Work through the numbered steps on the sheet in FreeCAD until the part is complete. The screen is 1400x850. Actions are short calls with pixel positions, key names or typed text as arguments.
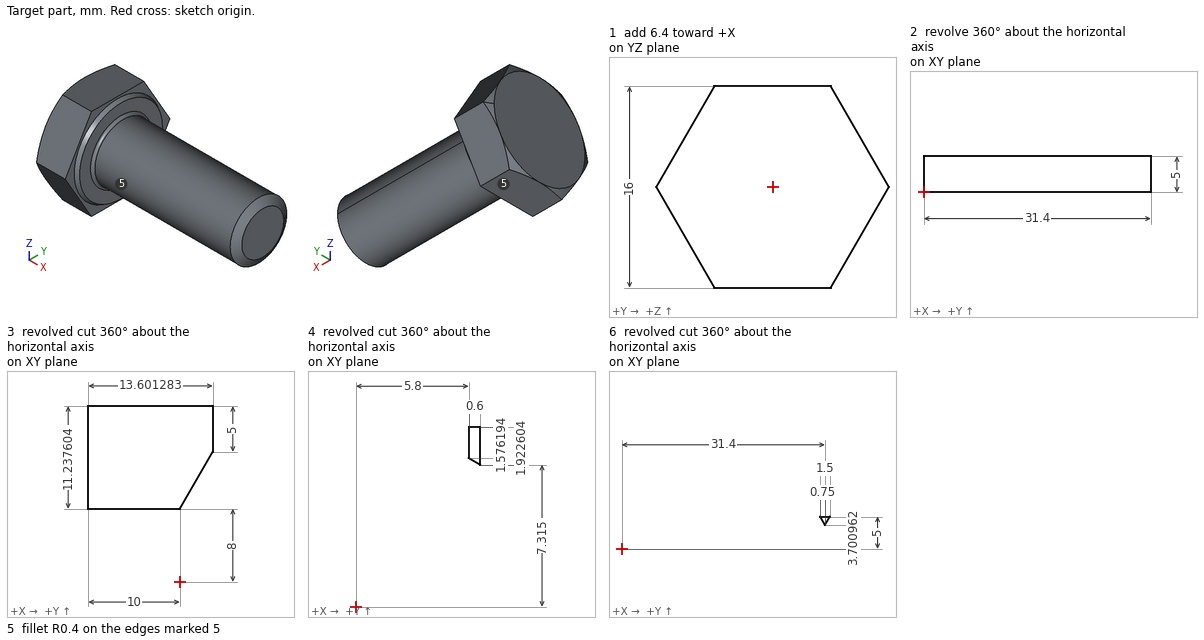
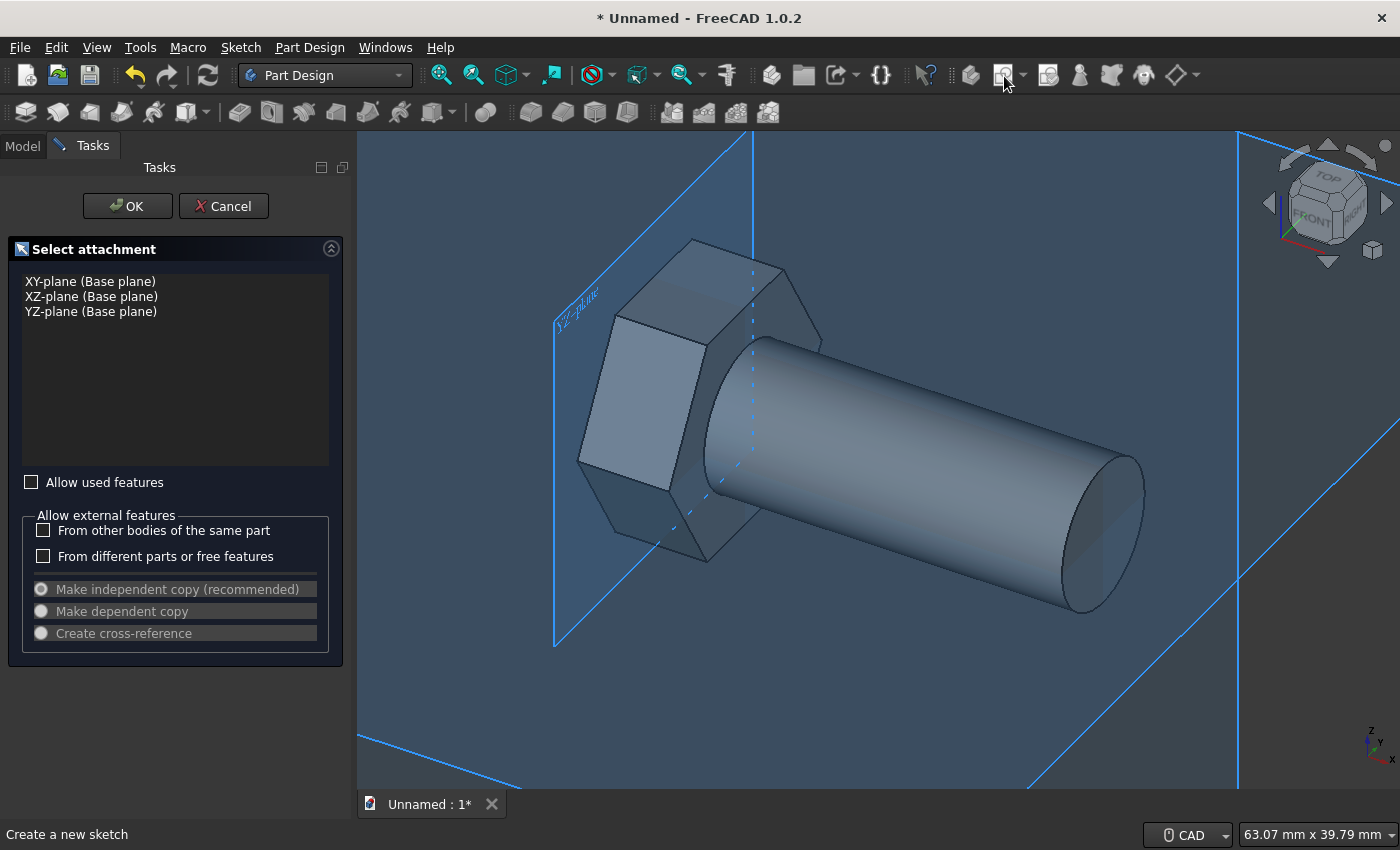
click(82, 282)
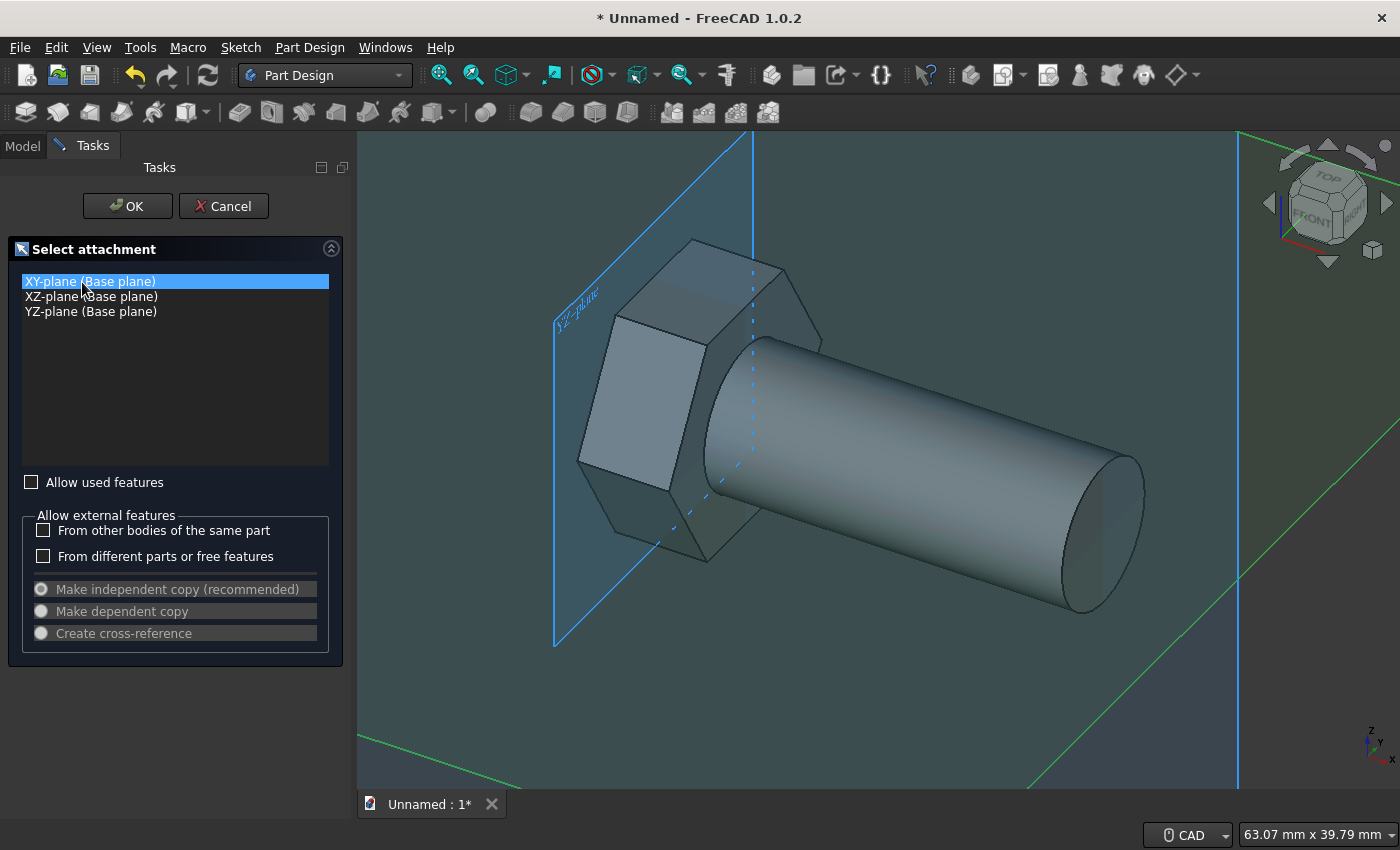
click(128, 206)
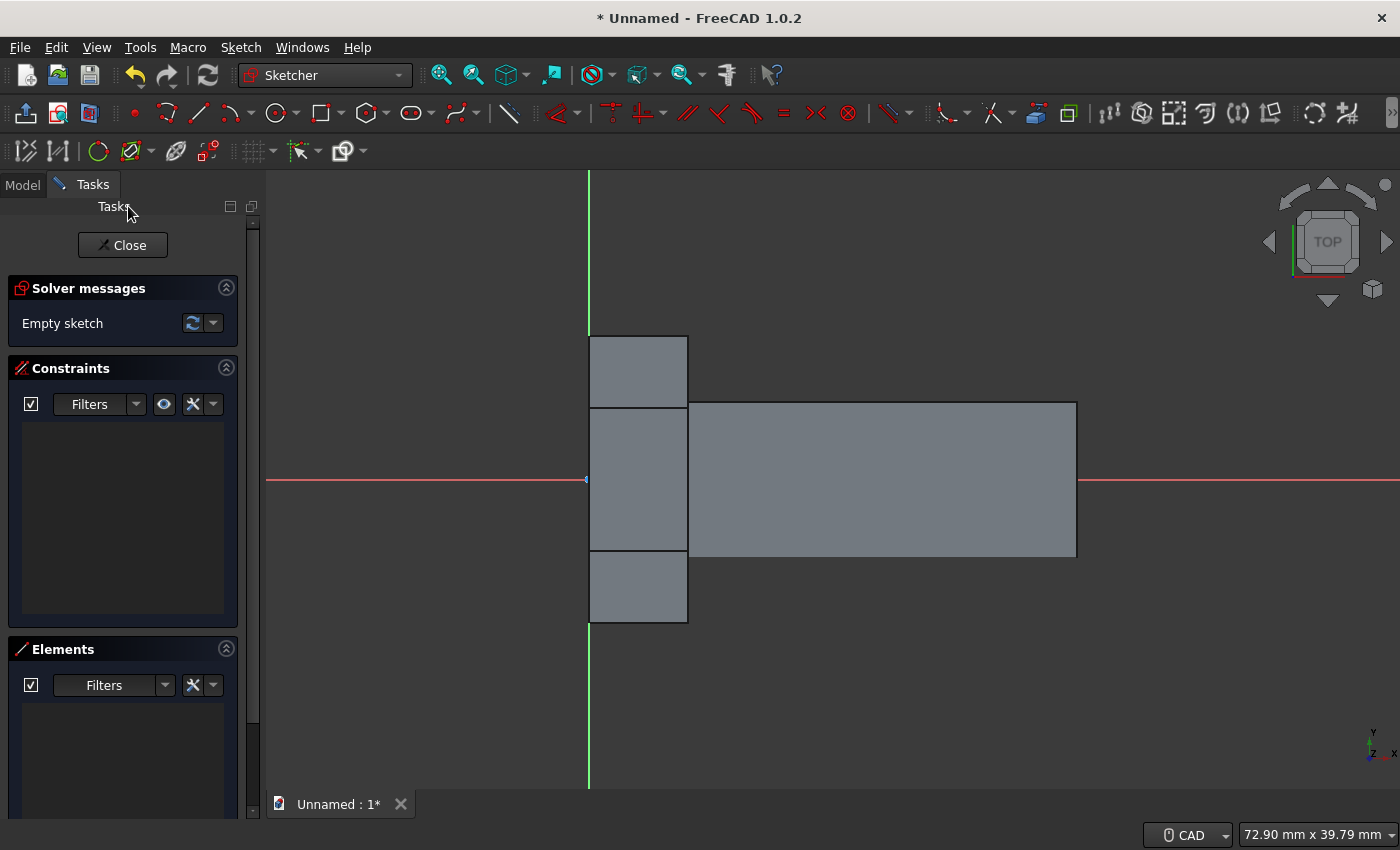
key(q)
key(s)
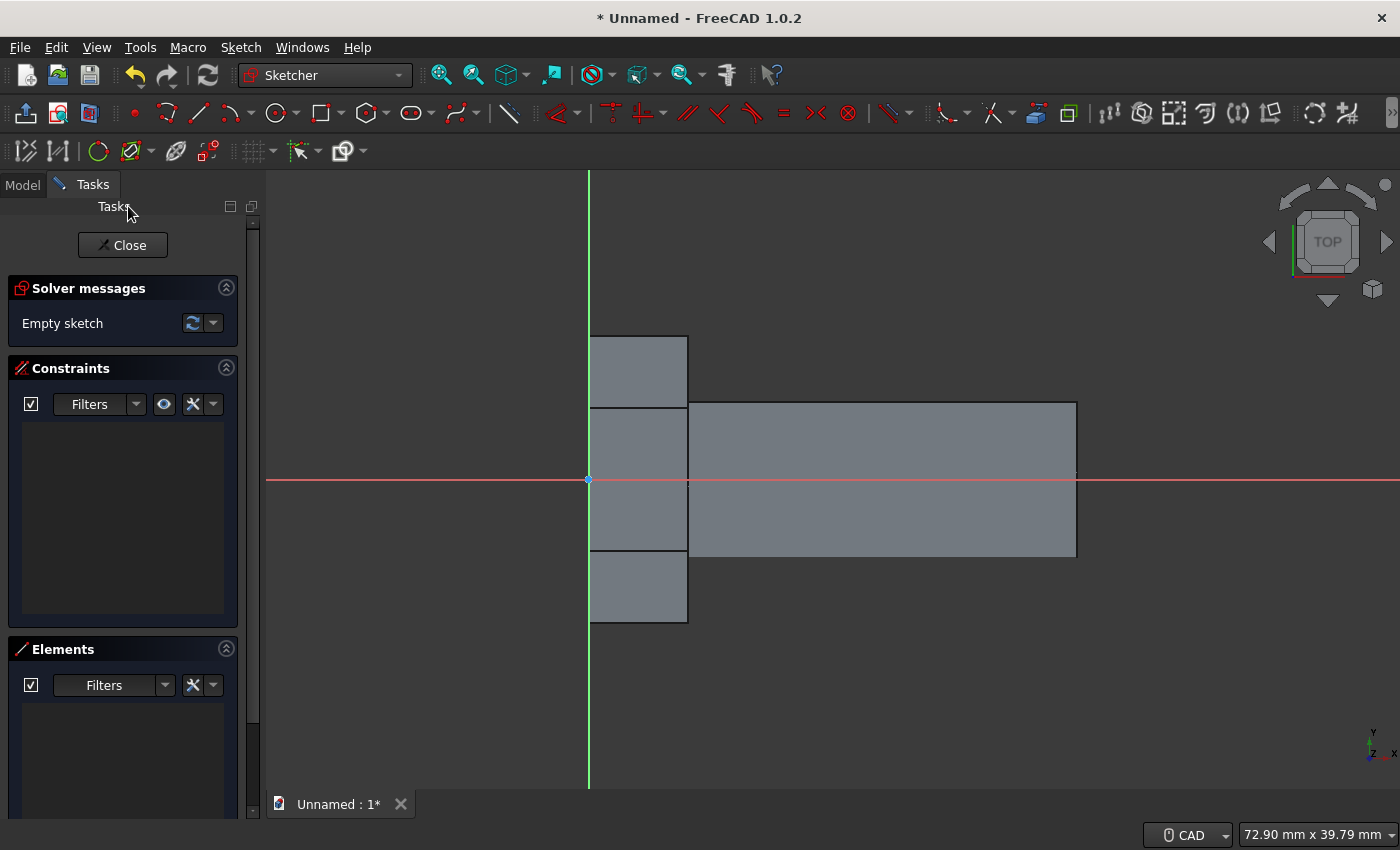
scroll(1235, 761, down, 1)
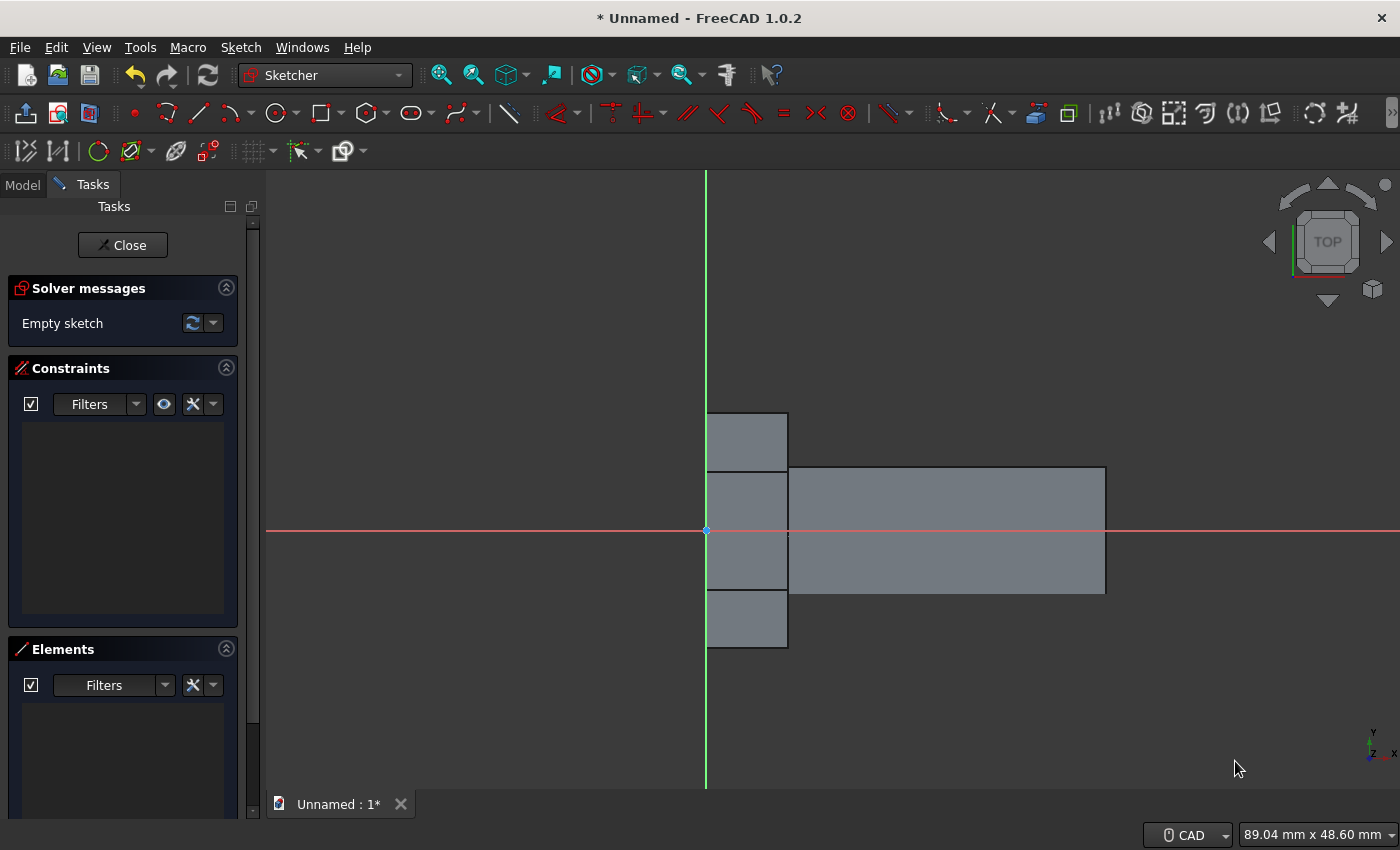
scroll(464, 263, up, 2)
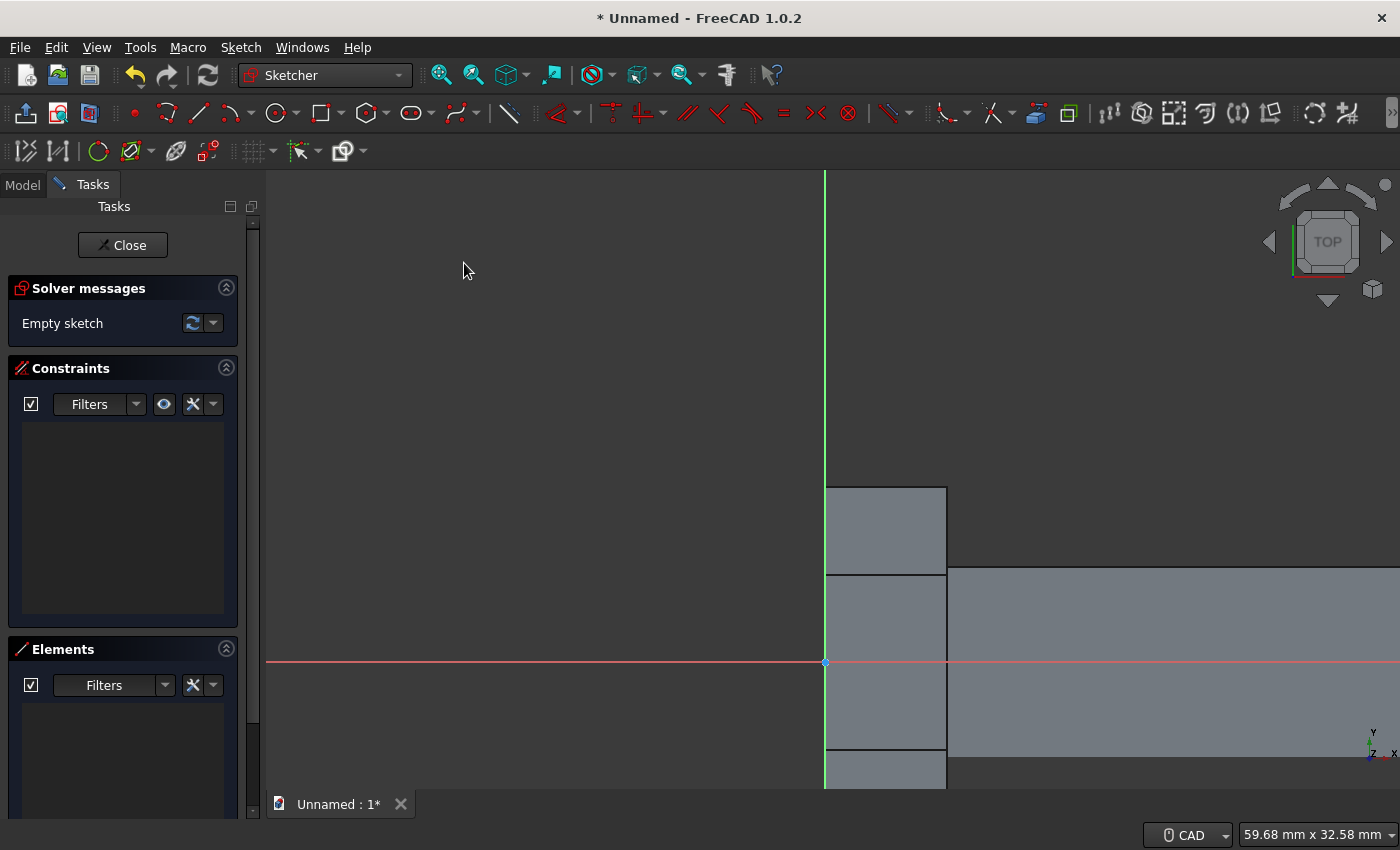
click(168, 114)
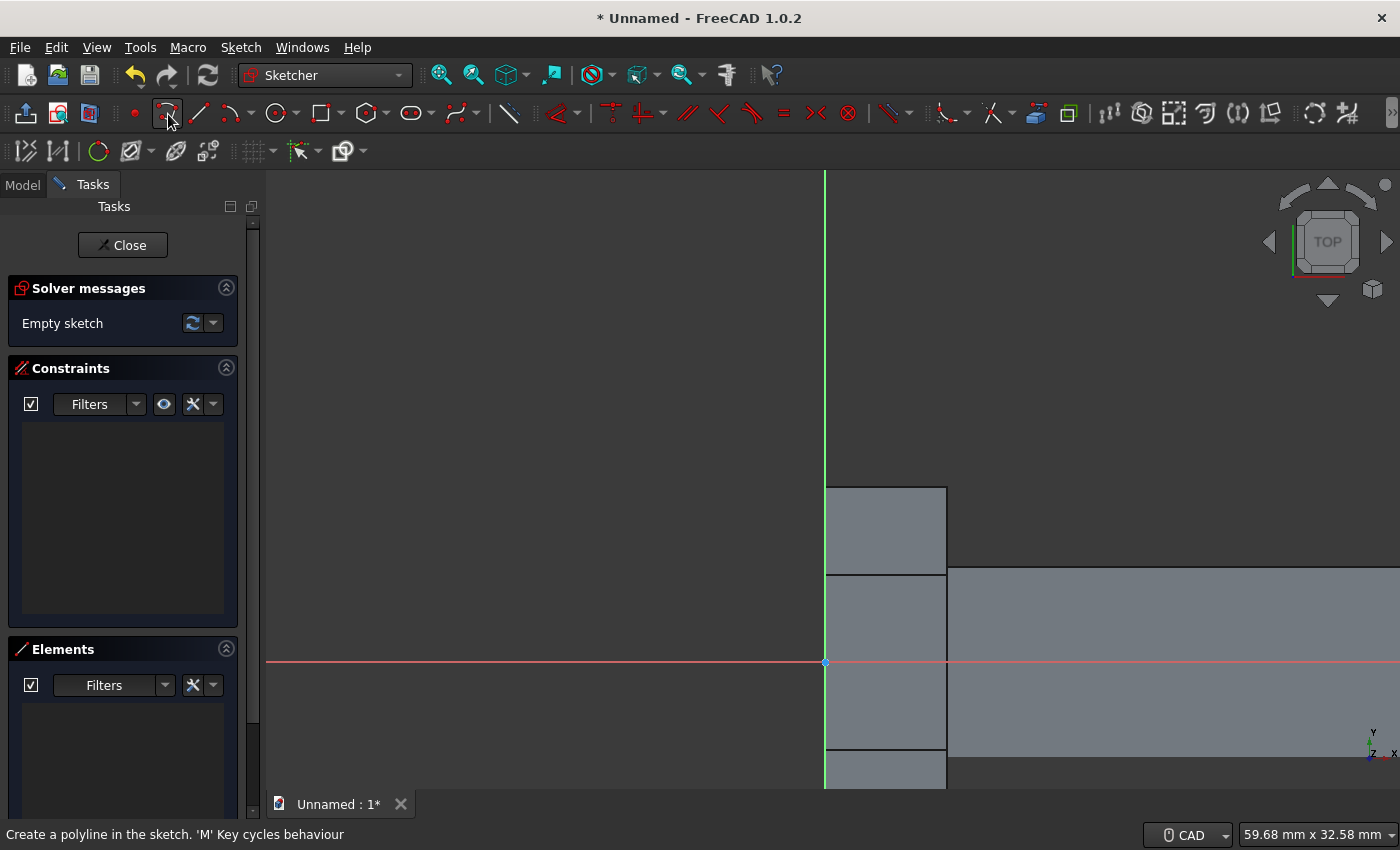
click(825, 510)
click(893, 392)
click(893, 297)
click(635, 297)
click(635, 510)
click(825, 511)
key(Escape)
key(Escape)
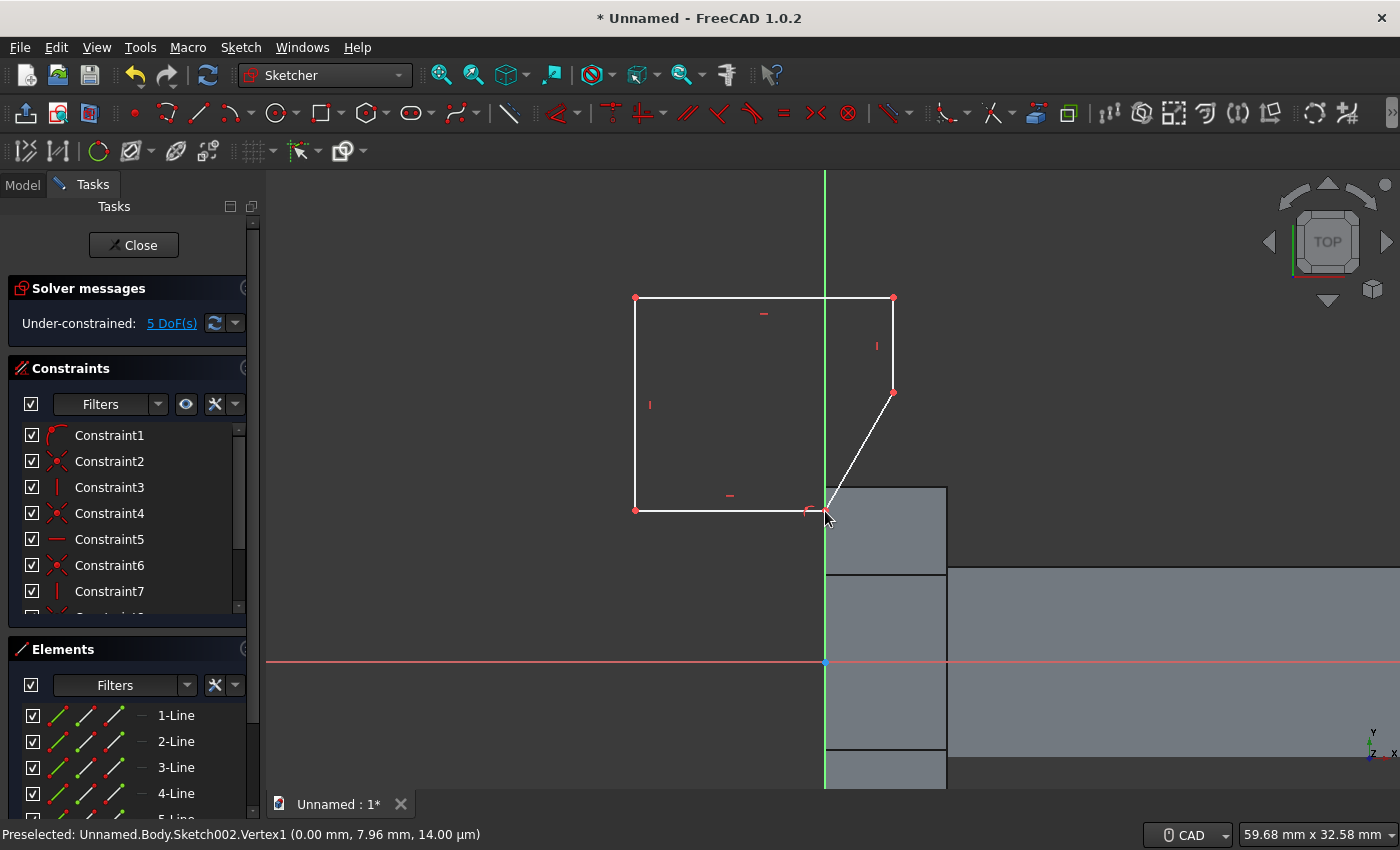
click(556, 114)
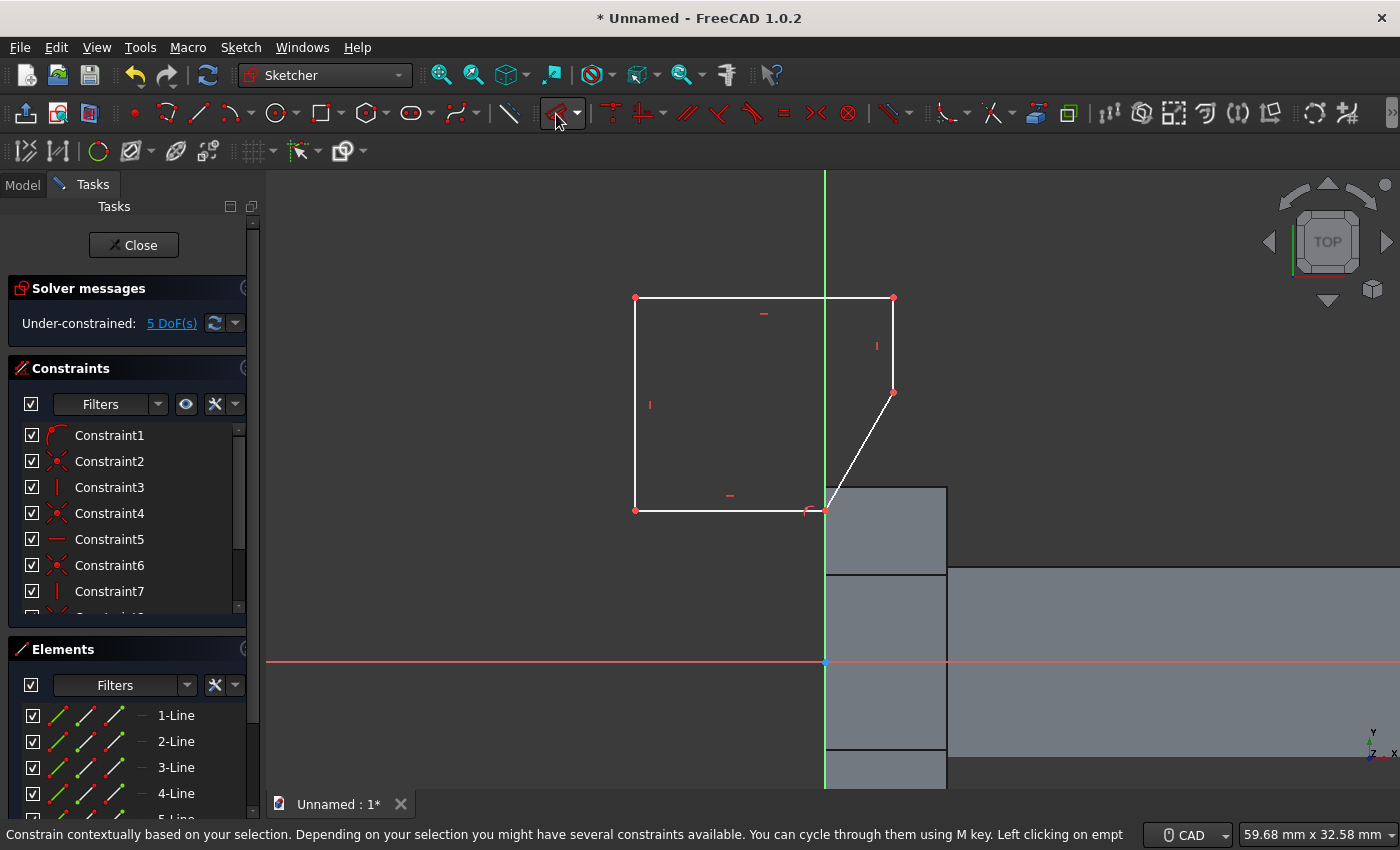
click(893, 365)
click(927, 346)